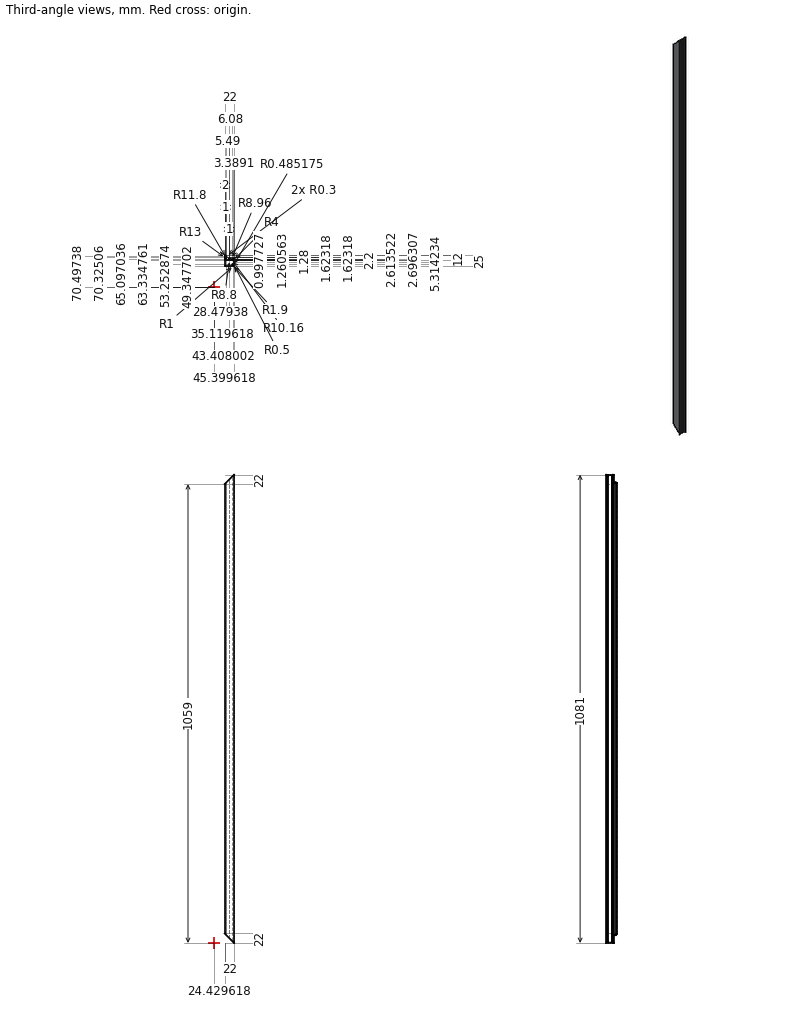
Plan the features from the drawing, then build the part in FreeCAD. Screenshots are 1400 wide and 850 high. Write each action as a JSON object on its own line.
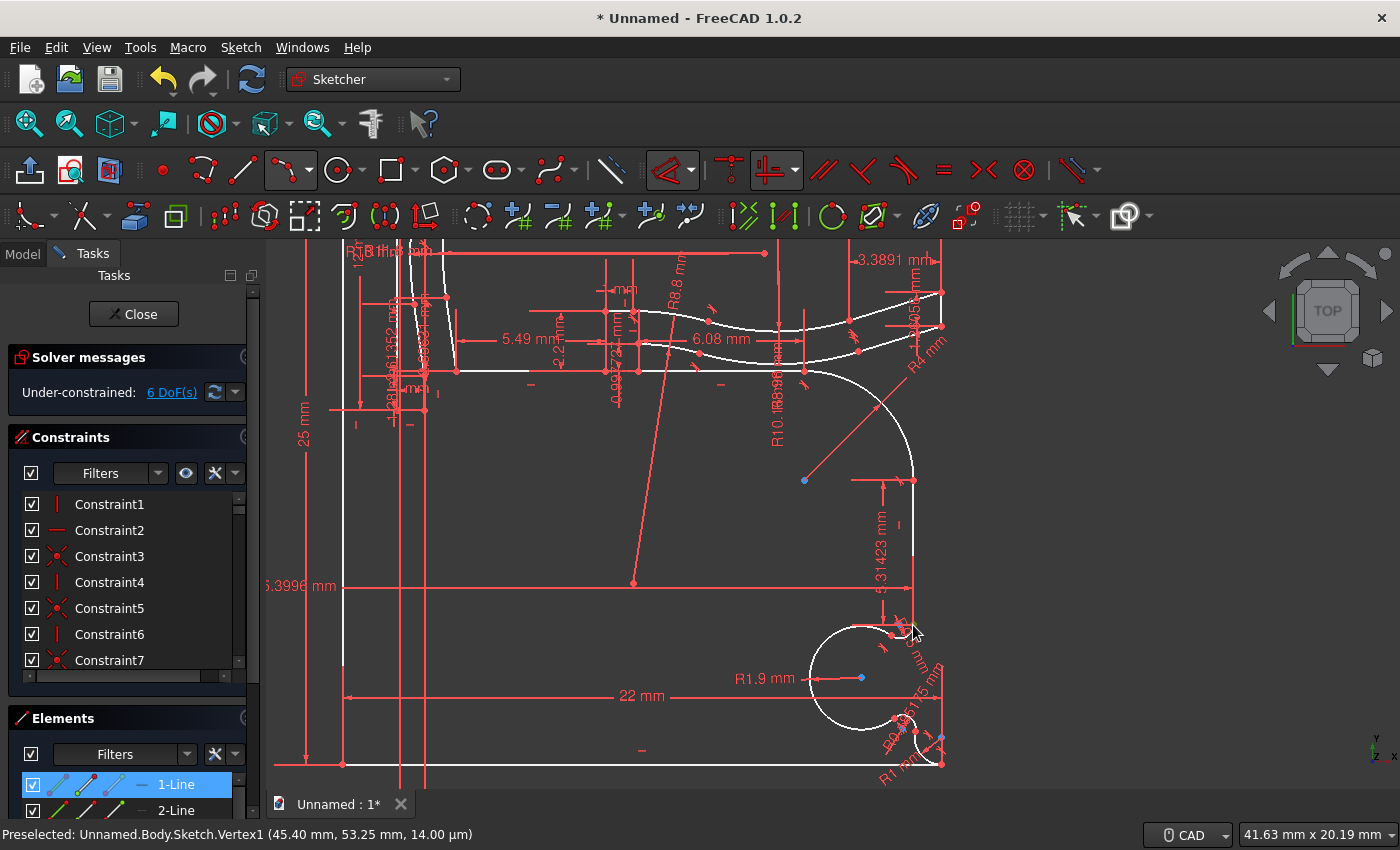
{"action": "left_click", "coordinate": [694, 170]}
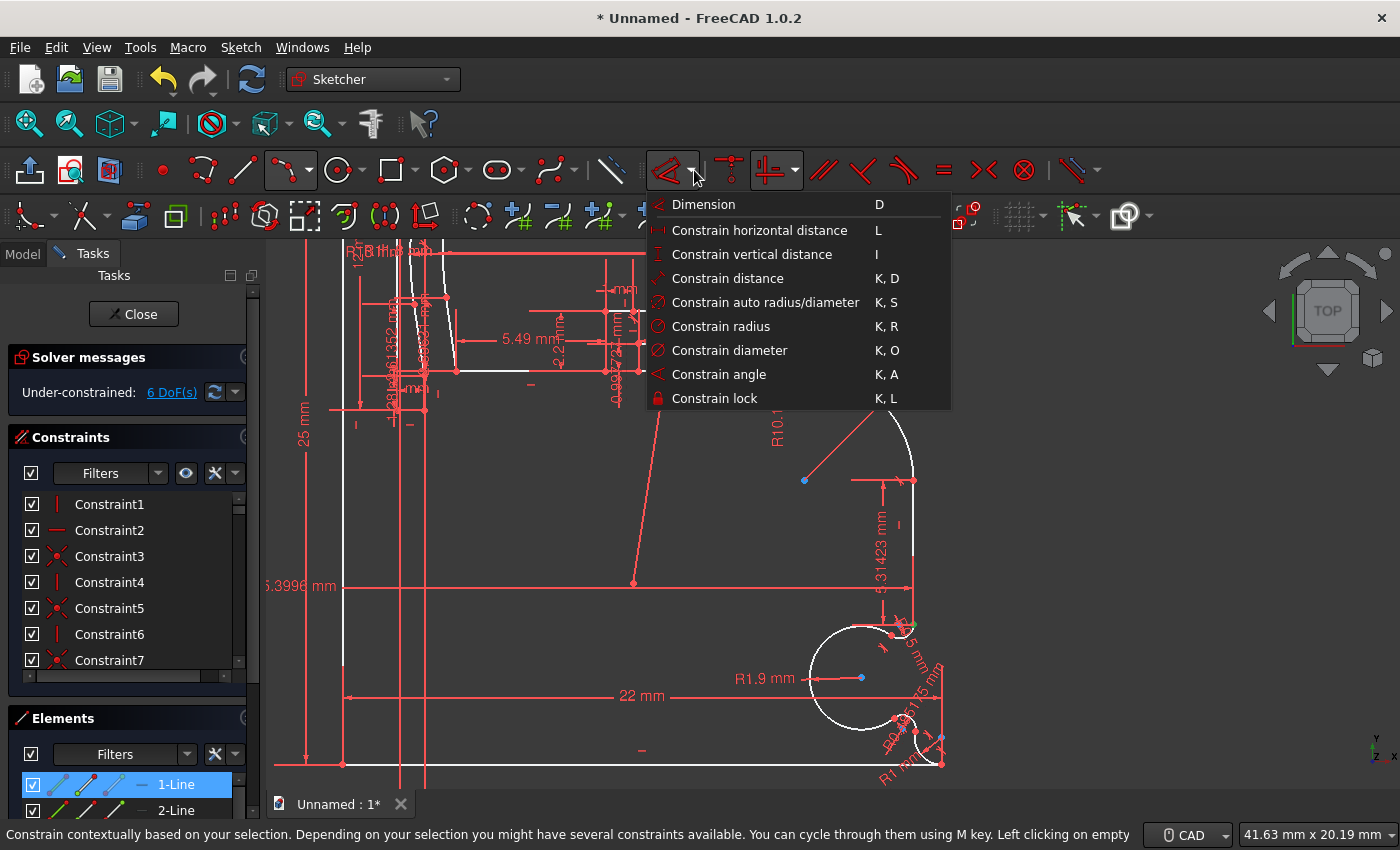
{"action": "left_click", "coordinate": [799, 254]}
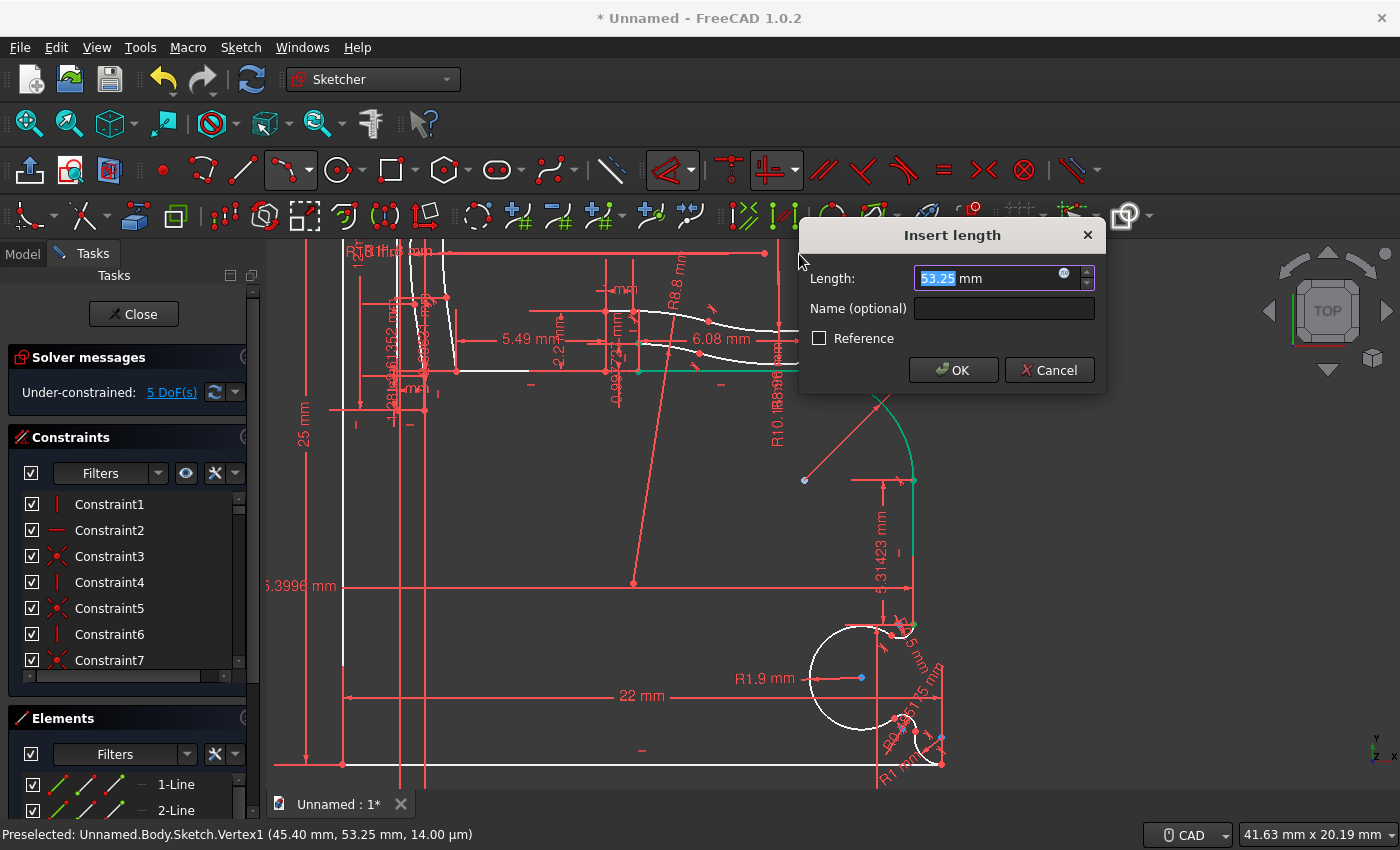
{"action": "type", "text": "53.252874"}
{"action": "key", "text": "Return"}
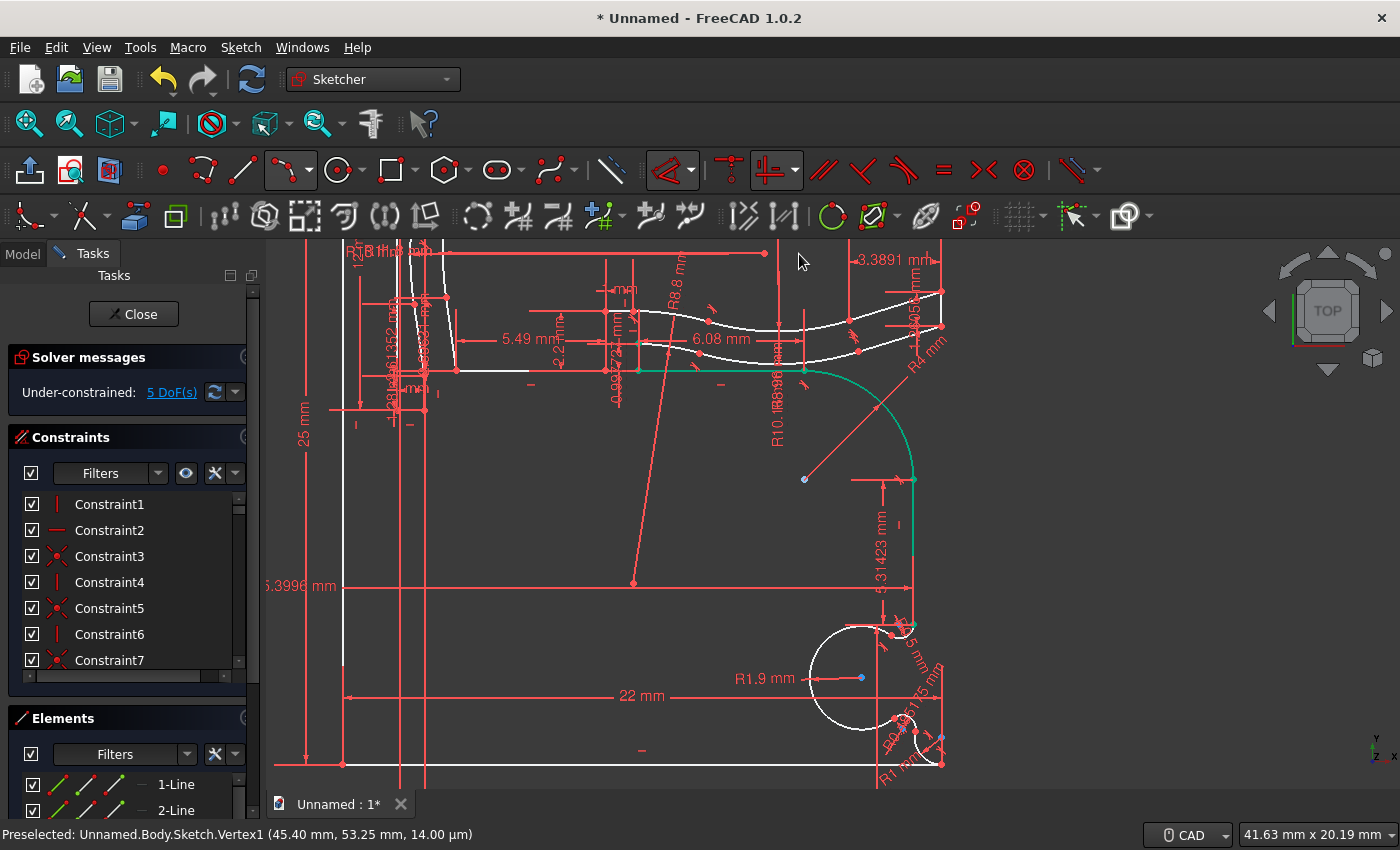
{"action": "left_click", "coordinate": [858, 352]}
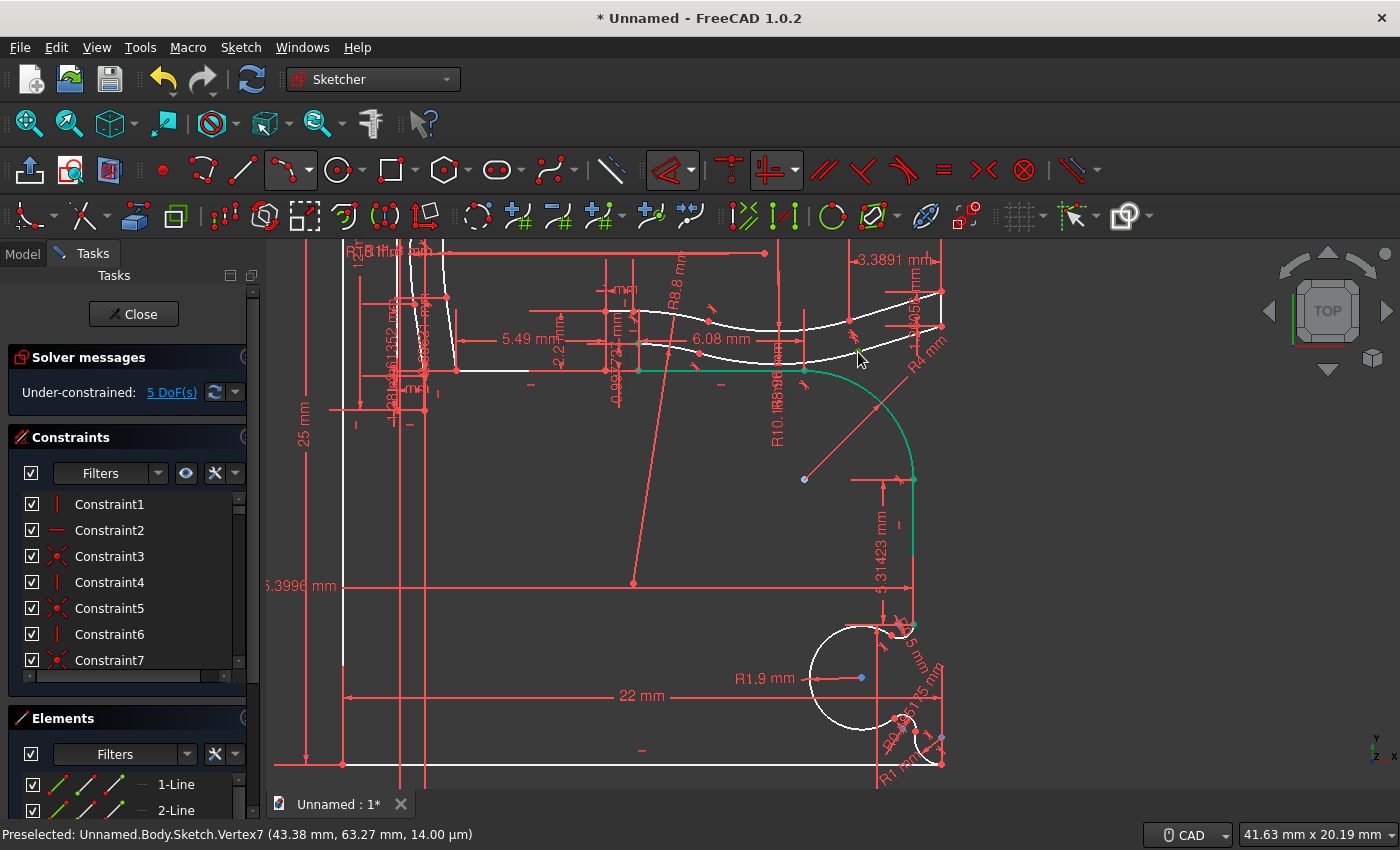
{"action": "key", "text": "l"}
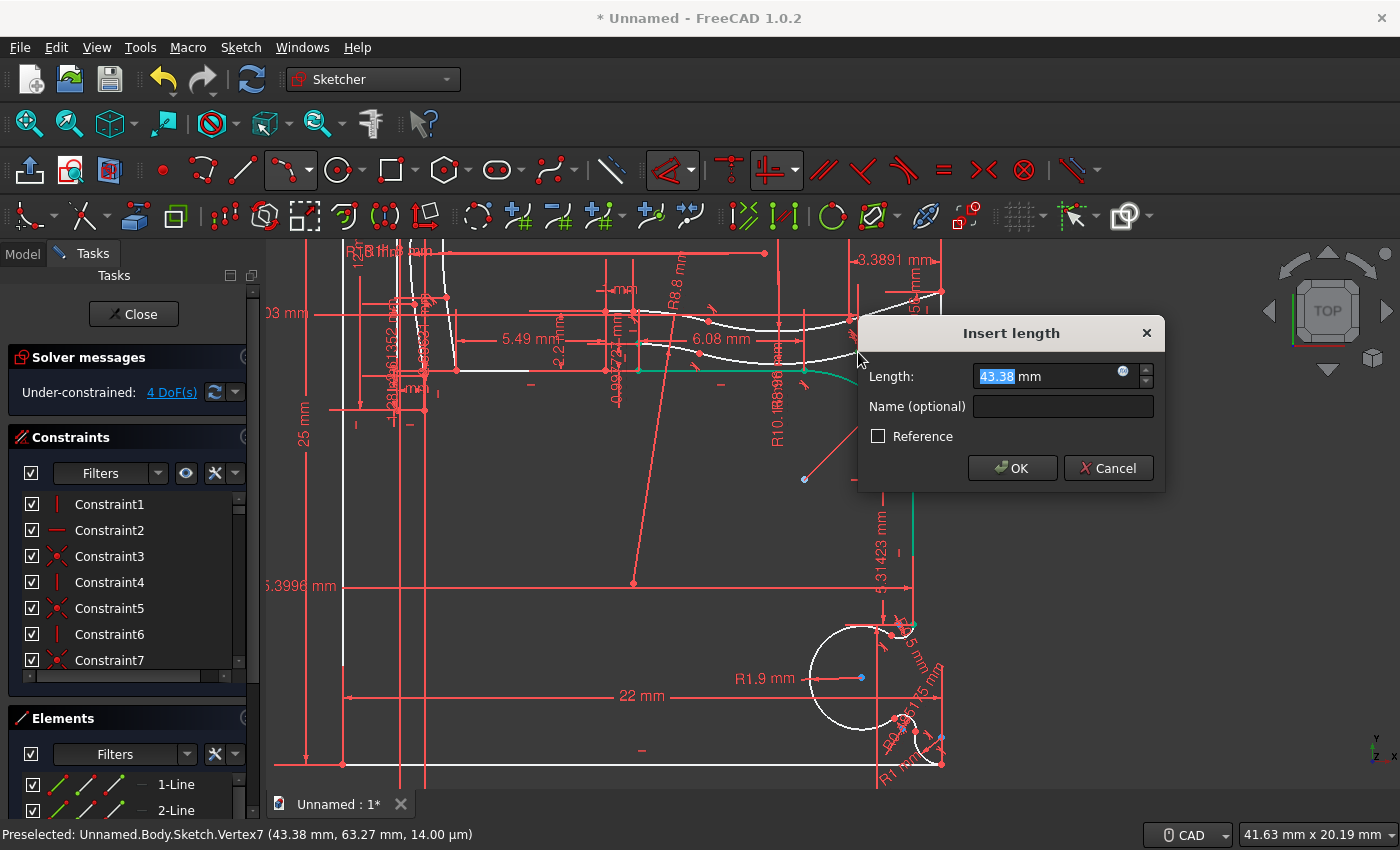
{"action": "type", "text": "43.408002"}
{"action": "key", "text": "Return"}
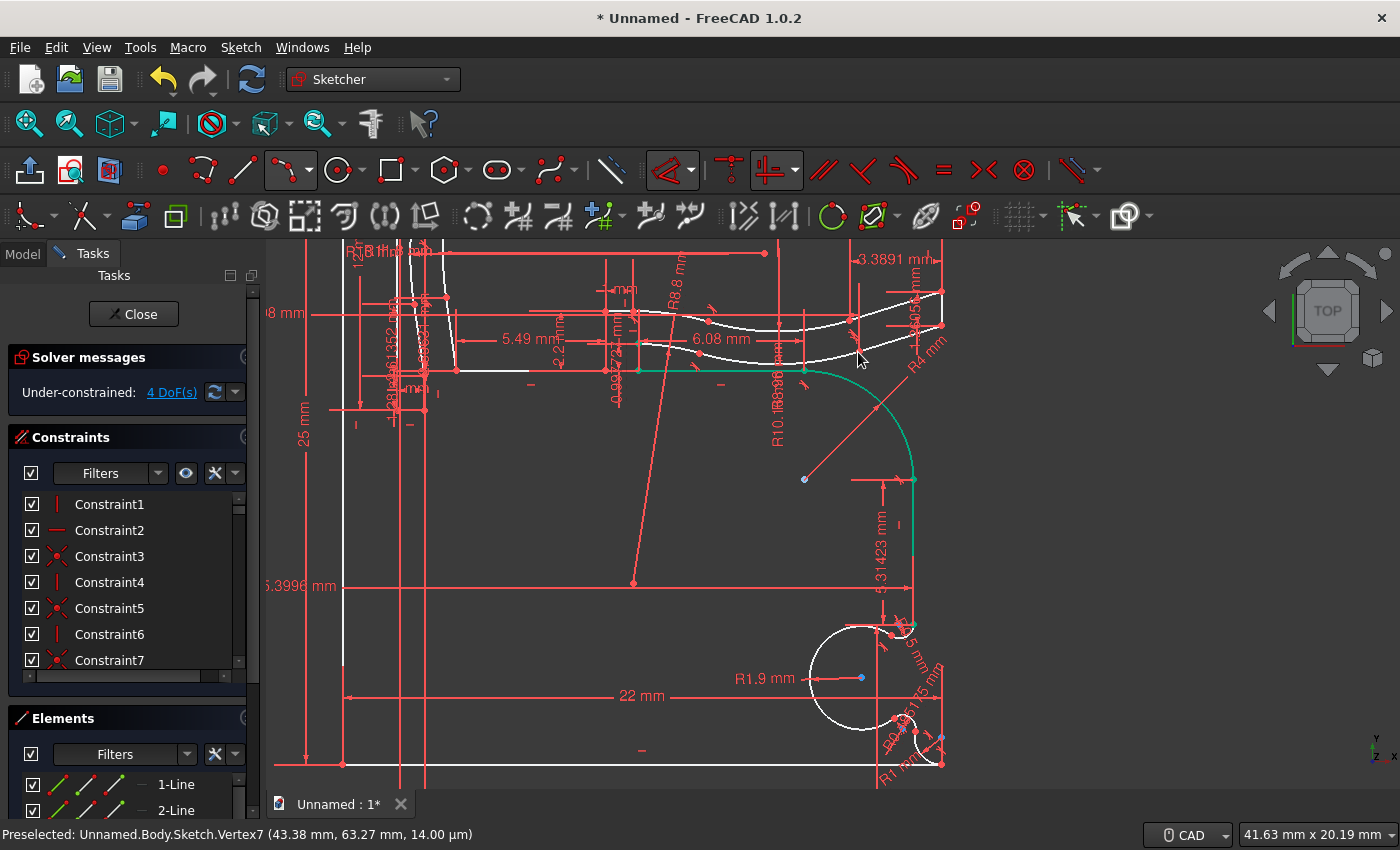
{"action": "left_click", "coordinate": [859, 352]}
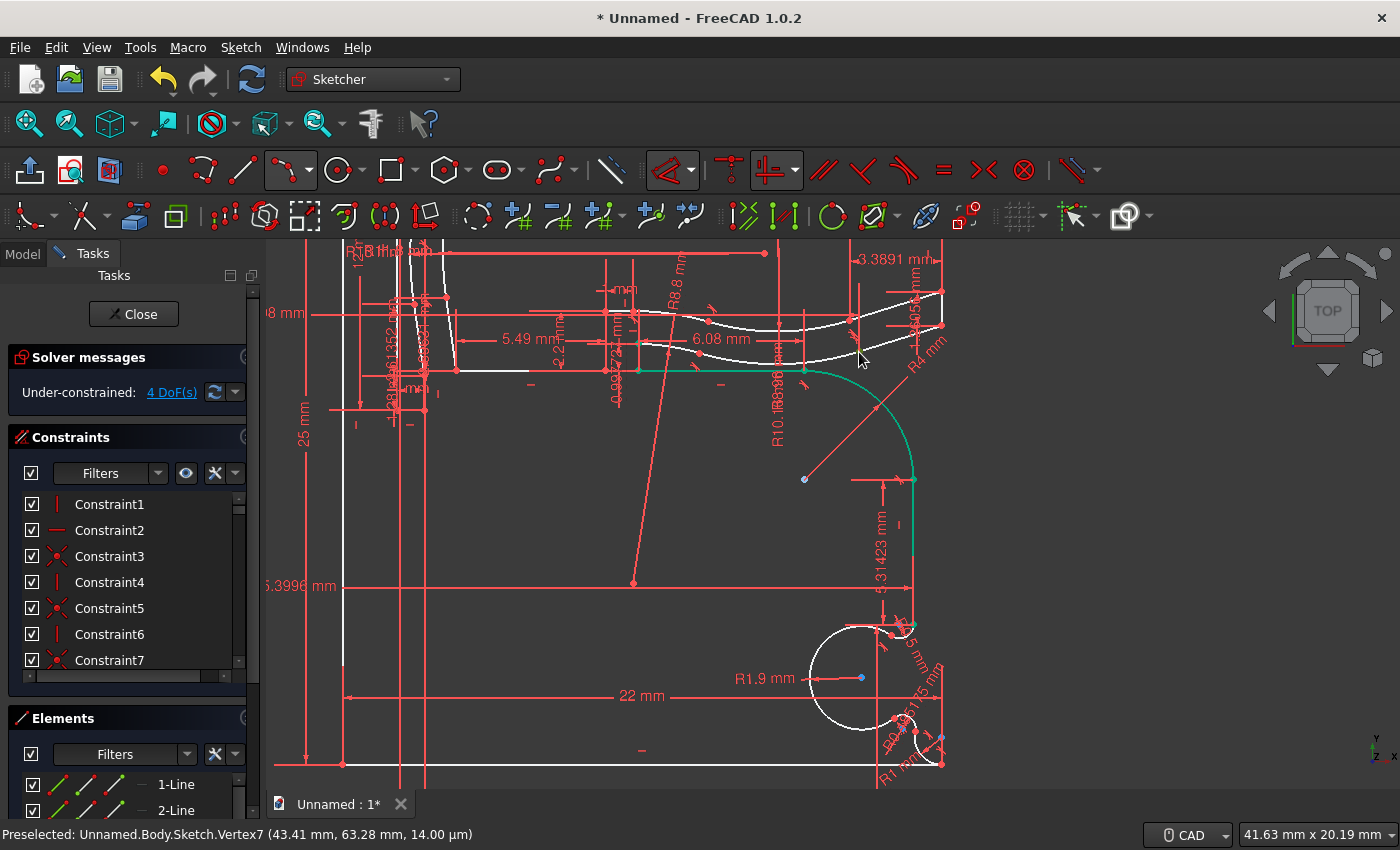
{"action": "key", "text": "i"}